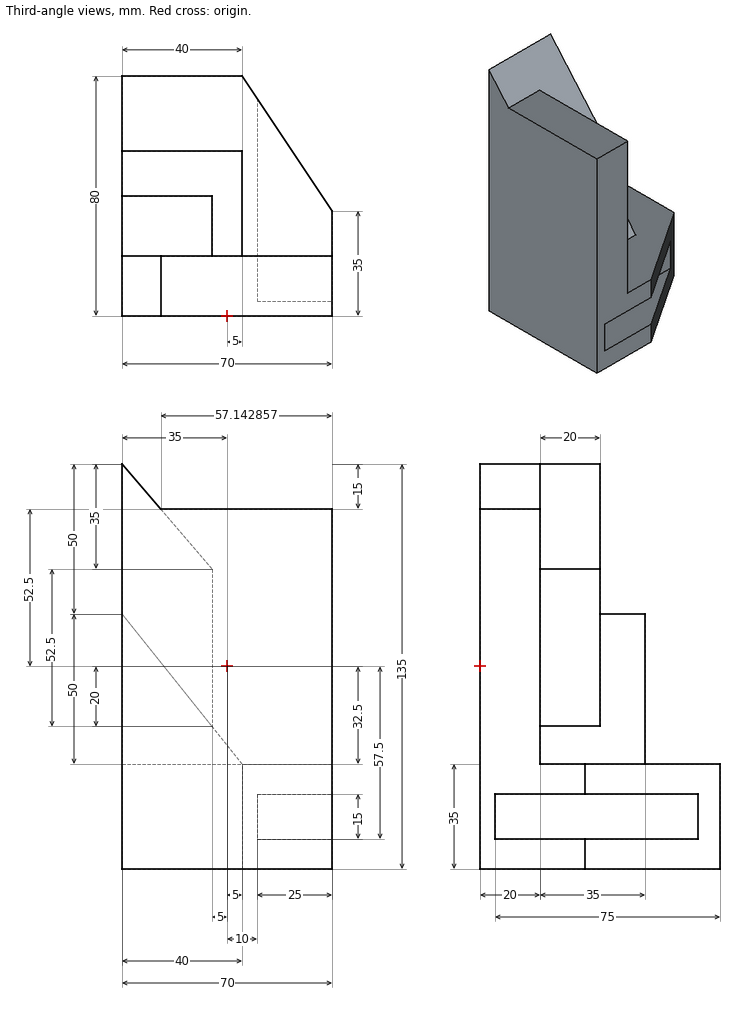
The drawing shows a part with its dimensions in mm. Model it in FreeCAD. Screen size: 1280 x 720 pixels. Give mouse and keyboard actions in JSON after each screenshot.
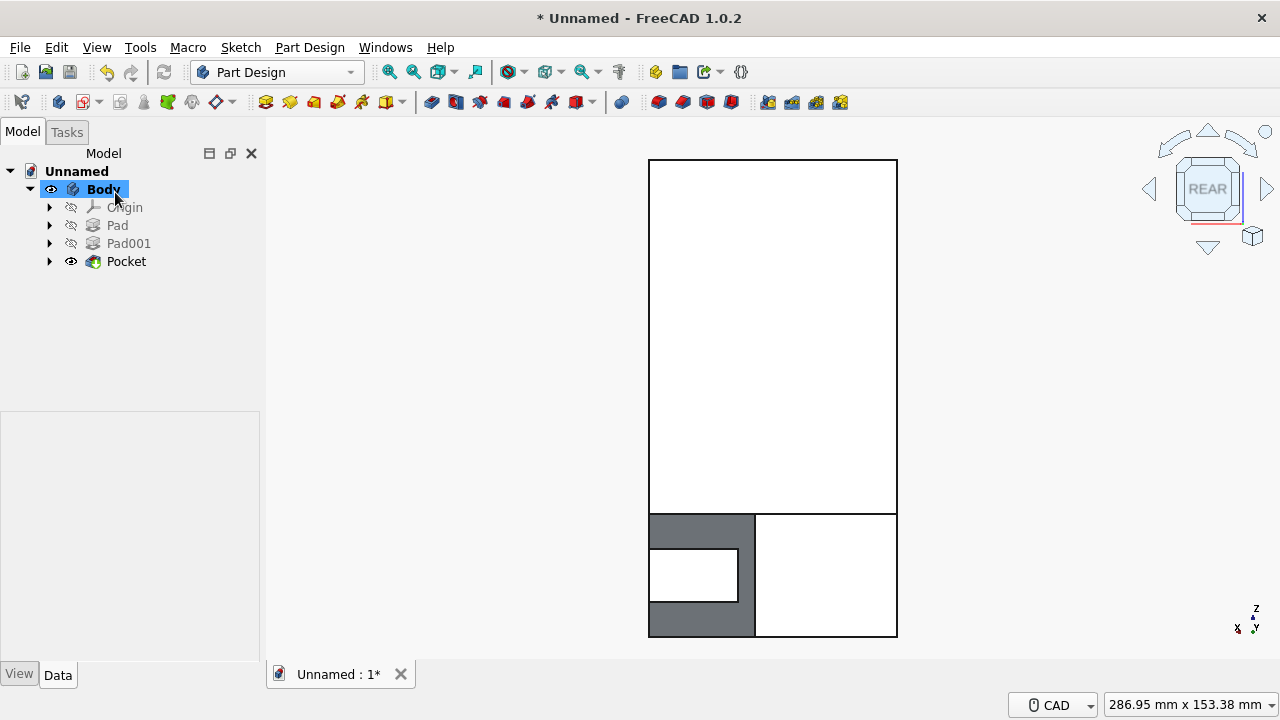
{"action": "left_click", "coordinate": [773, 285]}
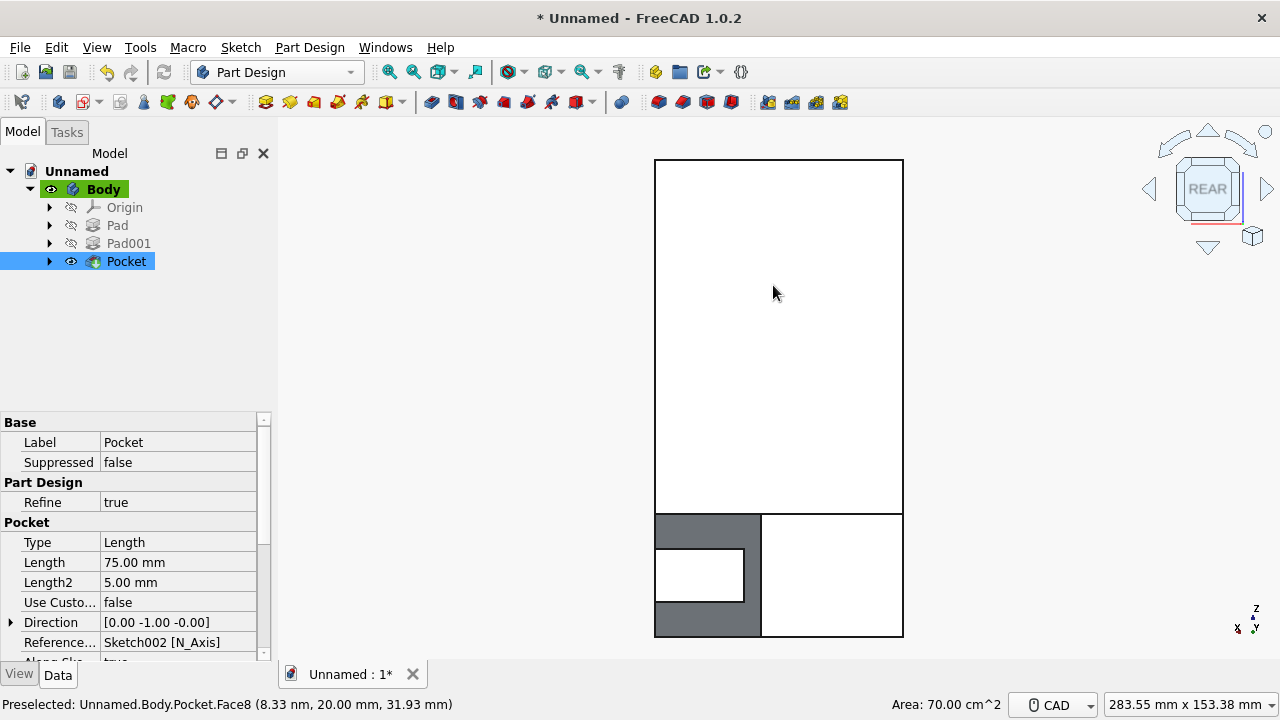
{"action": "left_click", "coordinate": [84, 102]}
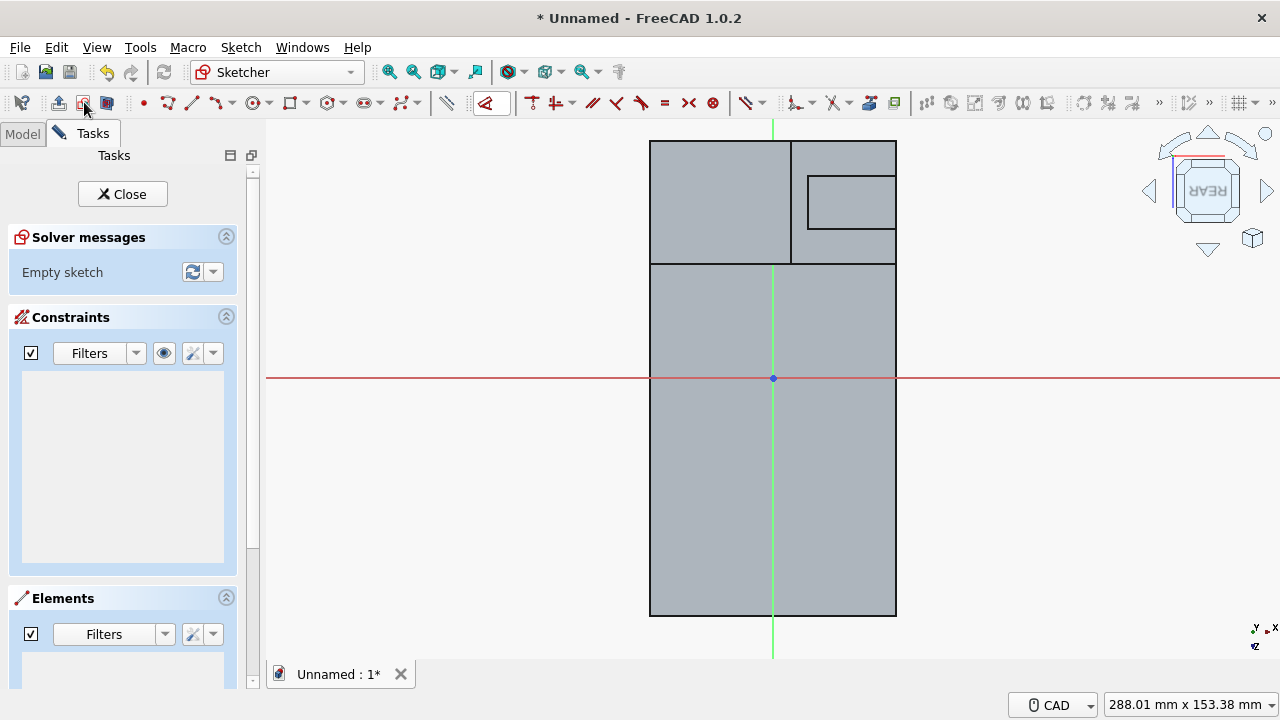
{"action": "scroll", "coordinate": [739, 307], "scroll_direction": "up", "scroll_amount": 3}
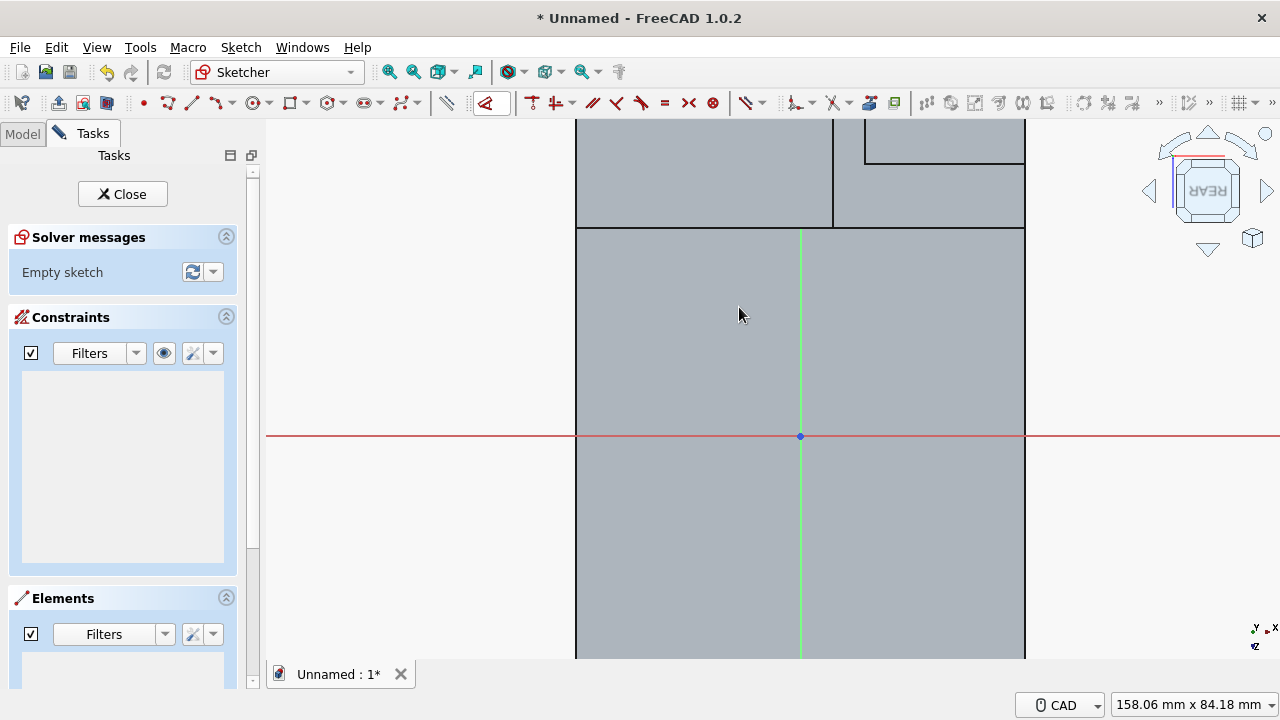
{"action": "left_click", "coordinate": [168, 104]}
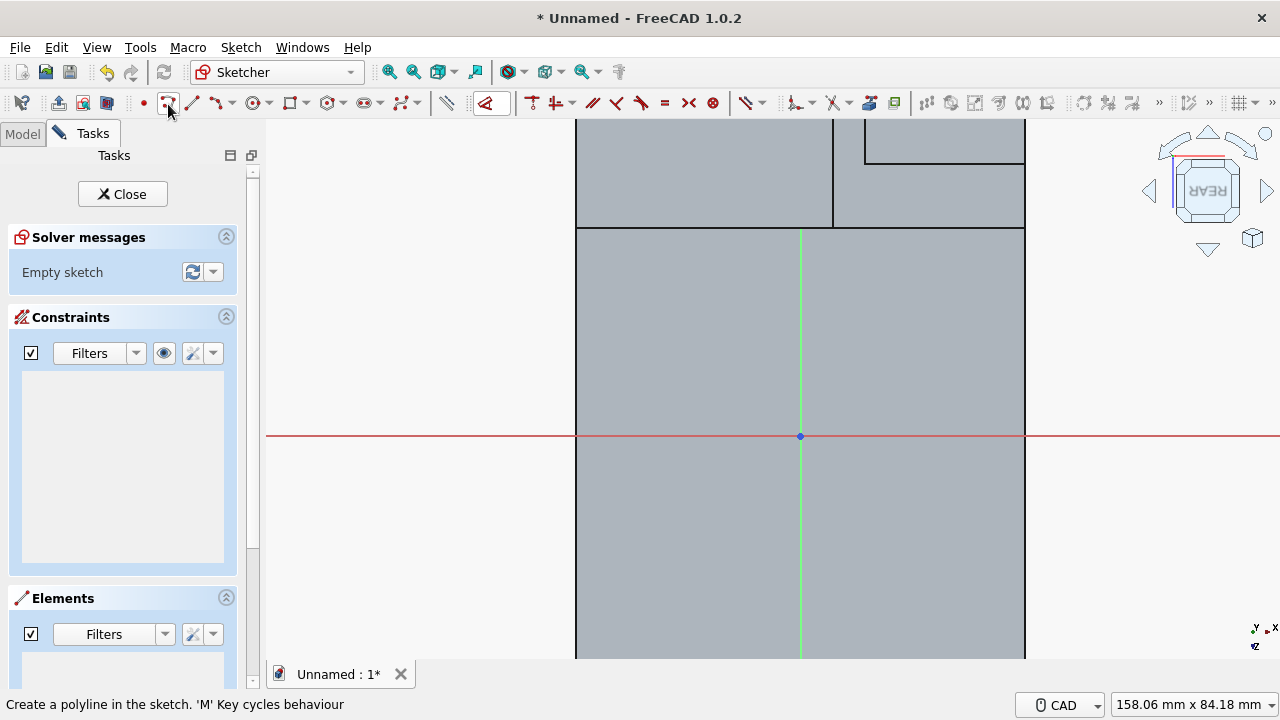
{"action": "left_click", "coordinate": [833, 228]}
{"action": "left_click", "coordinate": [576, 228]}
{"action": "left_click", "coordinate": [576, 549]}
{"action": "left_click", "coordinate": [833, 229]}
{"action": "key", "text": "Escape"}
{"action": "key", "text": "Escape"}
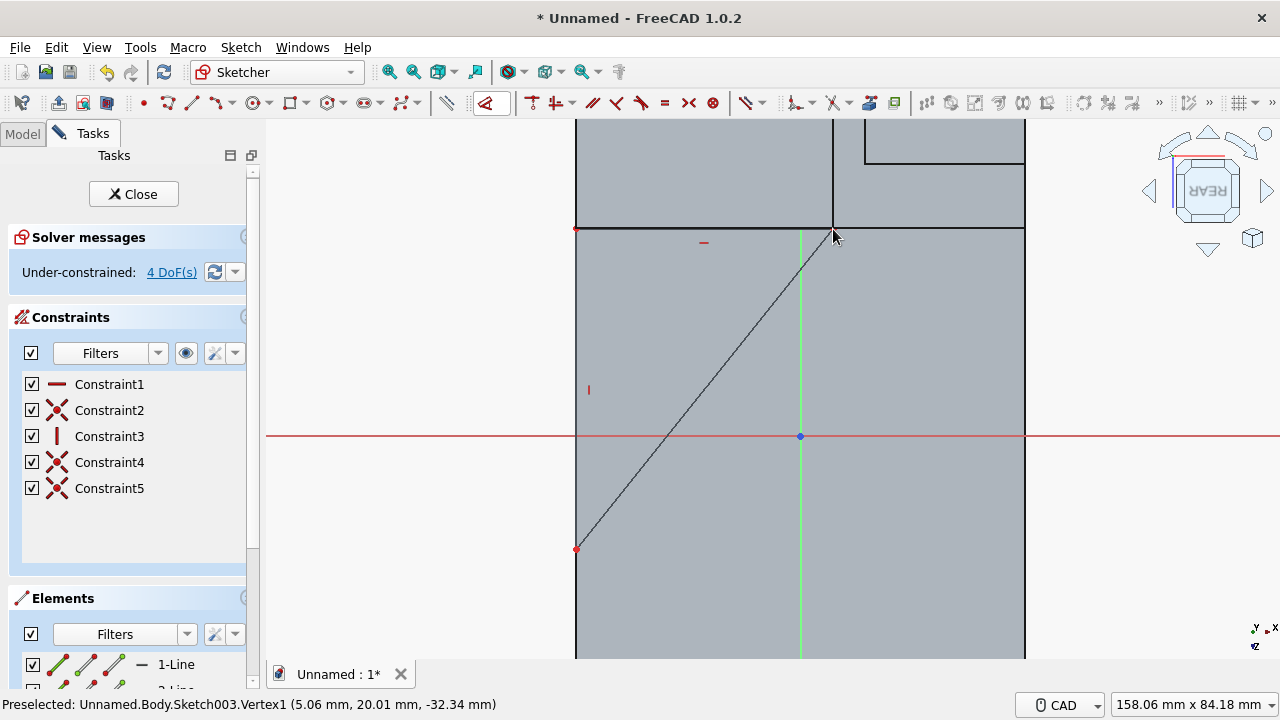
{"action": "left_click", "coordinate": [756, 229]}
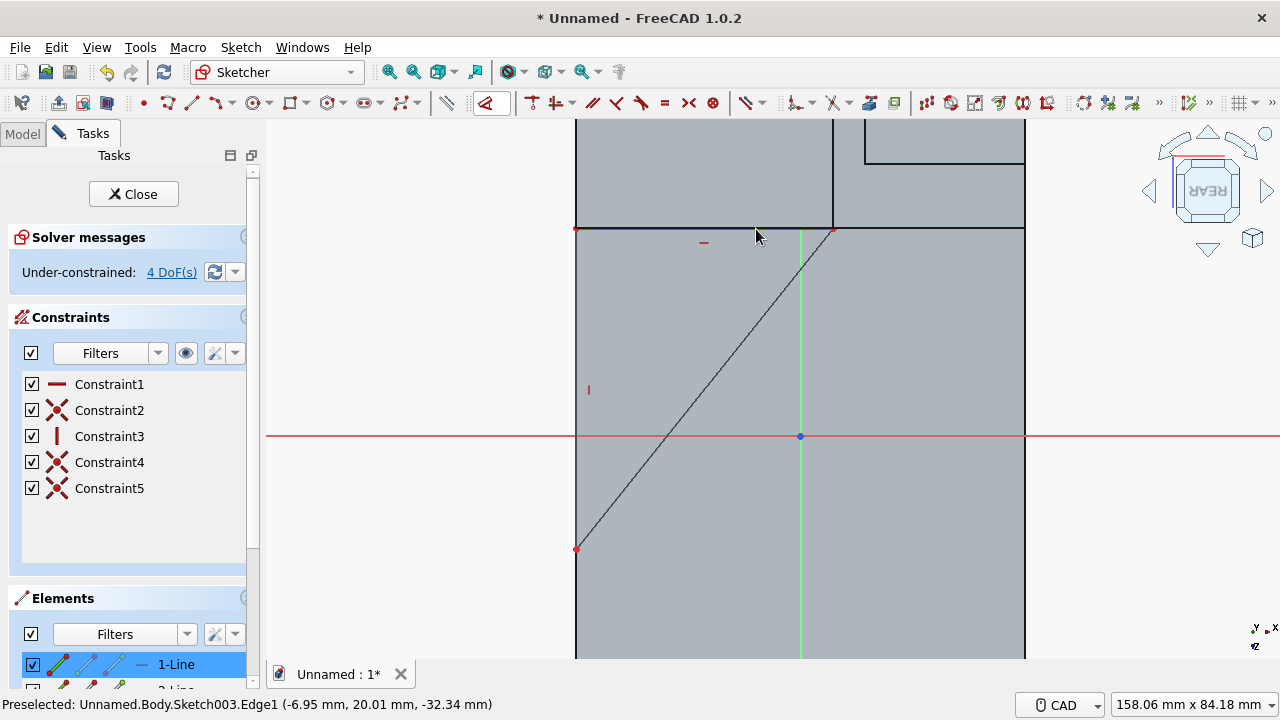
{"action": "left_click", "coordinate": [504, 104]}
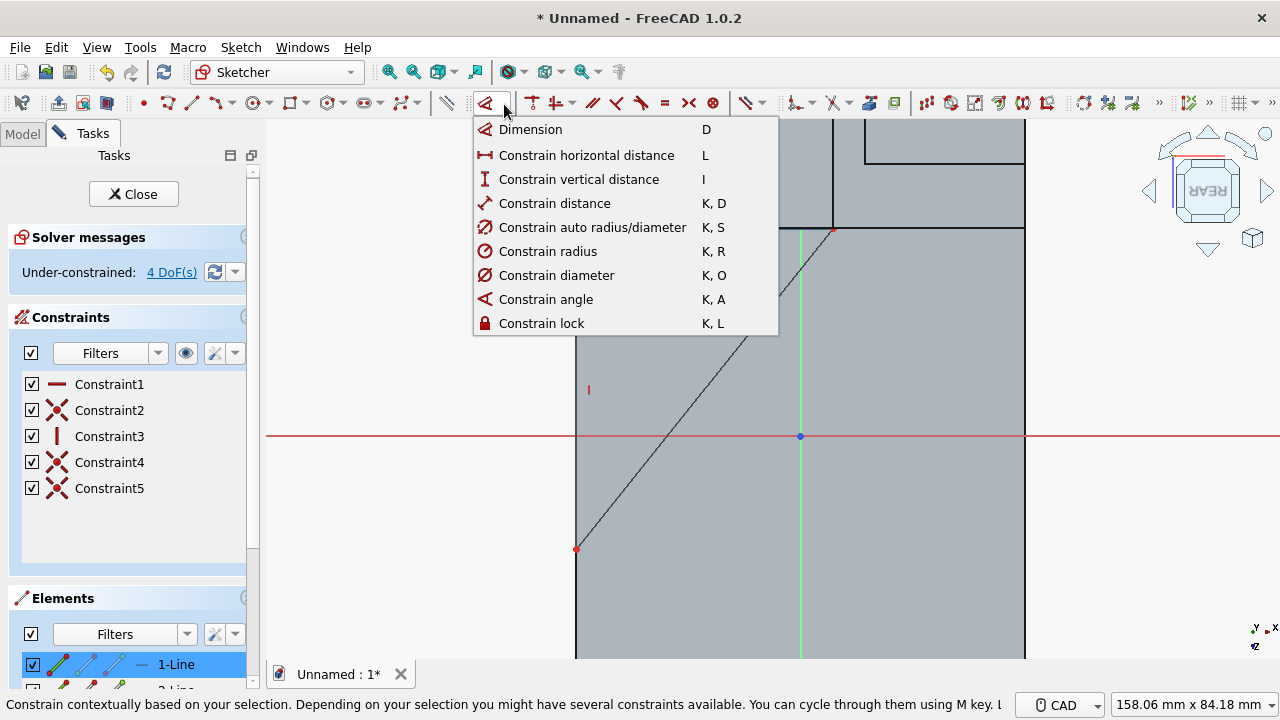
{"action": "left_click", "coordinate": [626, 155]}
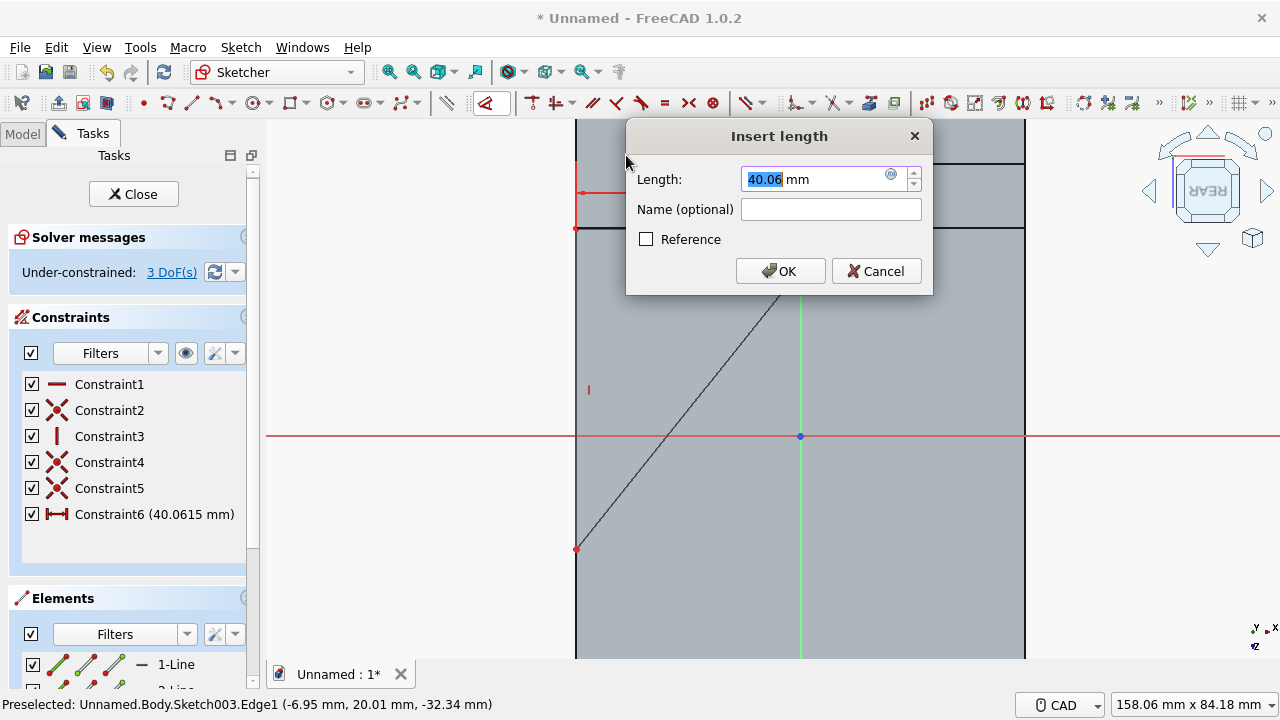
{"action": "type", "text": "40"}
{"action": "key", "text": "Return"}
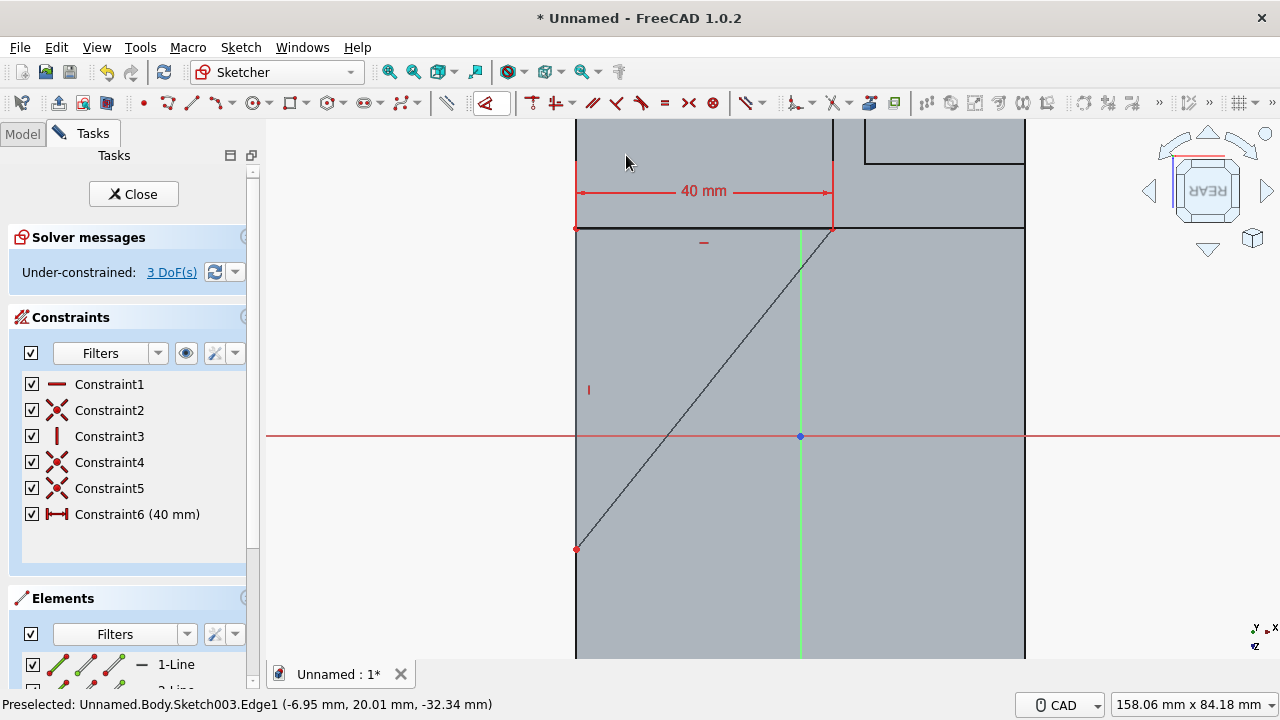
{"action": "left_click", "coordinate": [576, 325]}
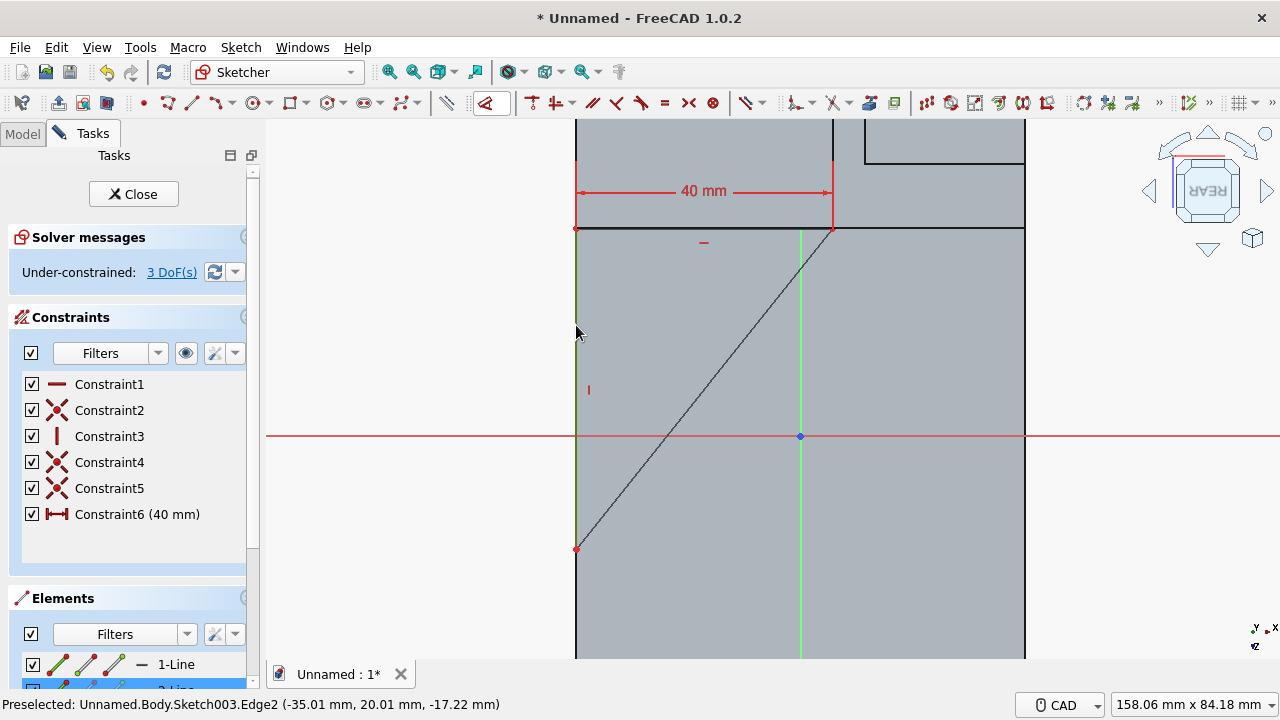
{"action": "key", "text": "i"}